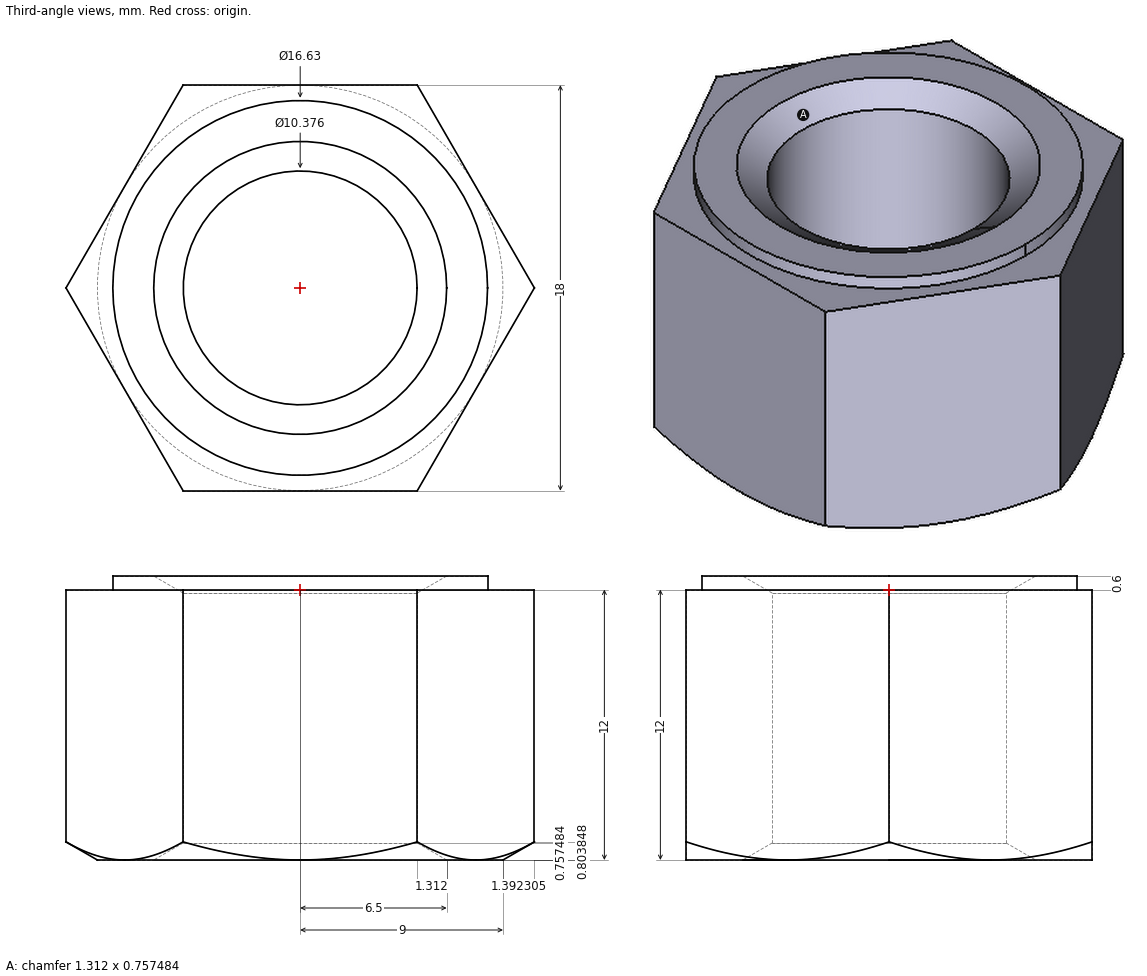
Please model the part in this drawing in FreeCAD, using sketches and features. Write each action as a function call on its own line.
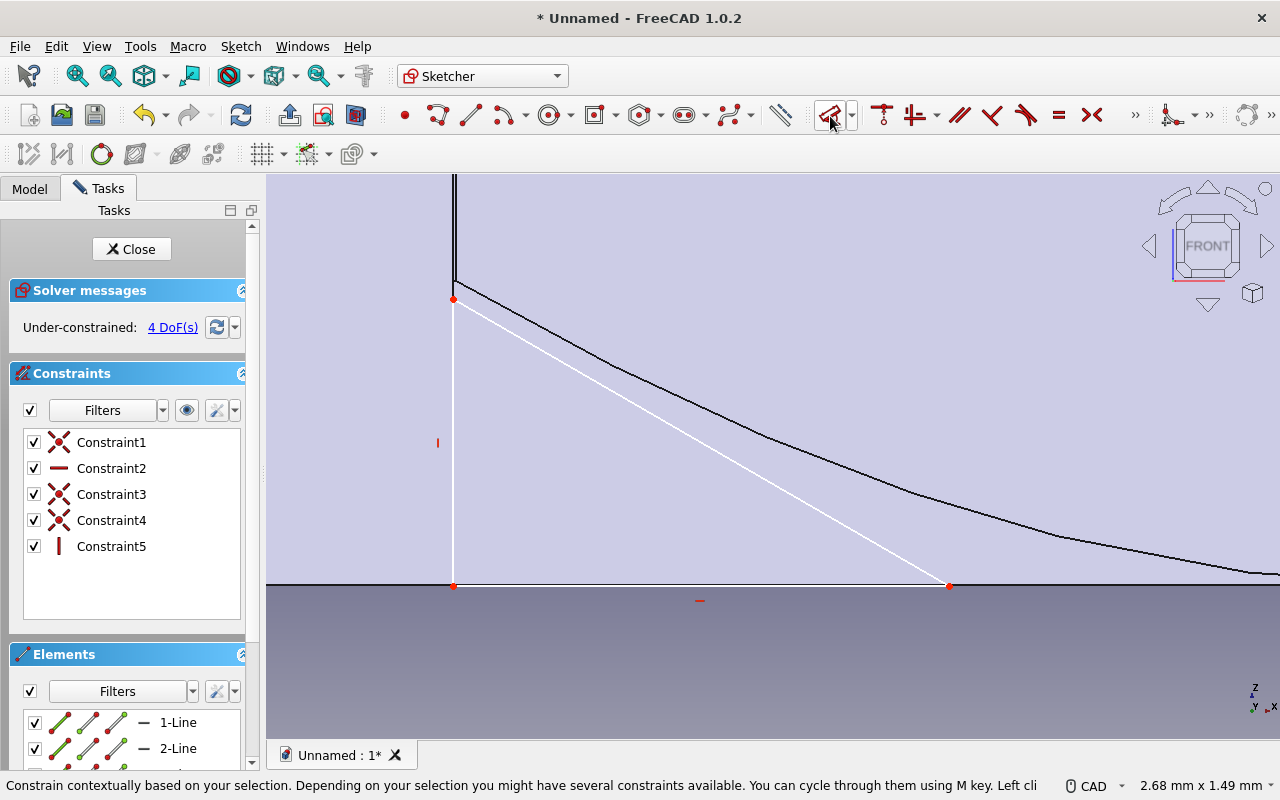
click(949, 586)
click(983, 394)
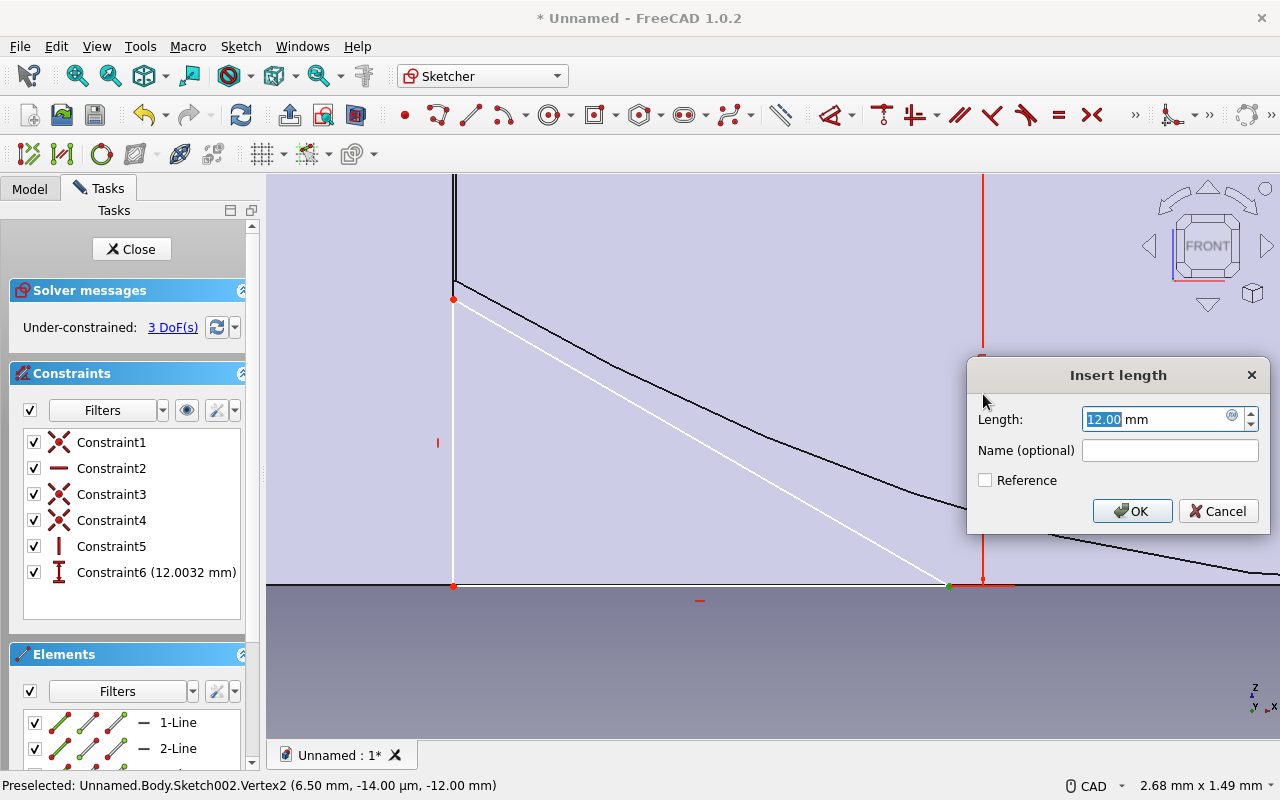
text(12)
key(Return)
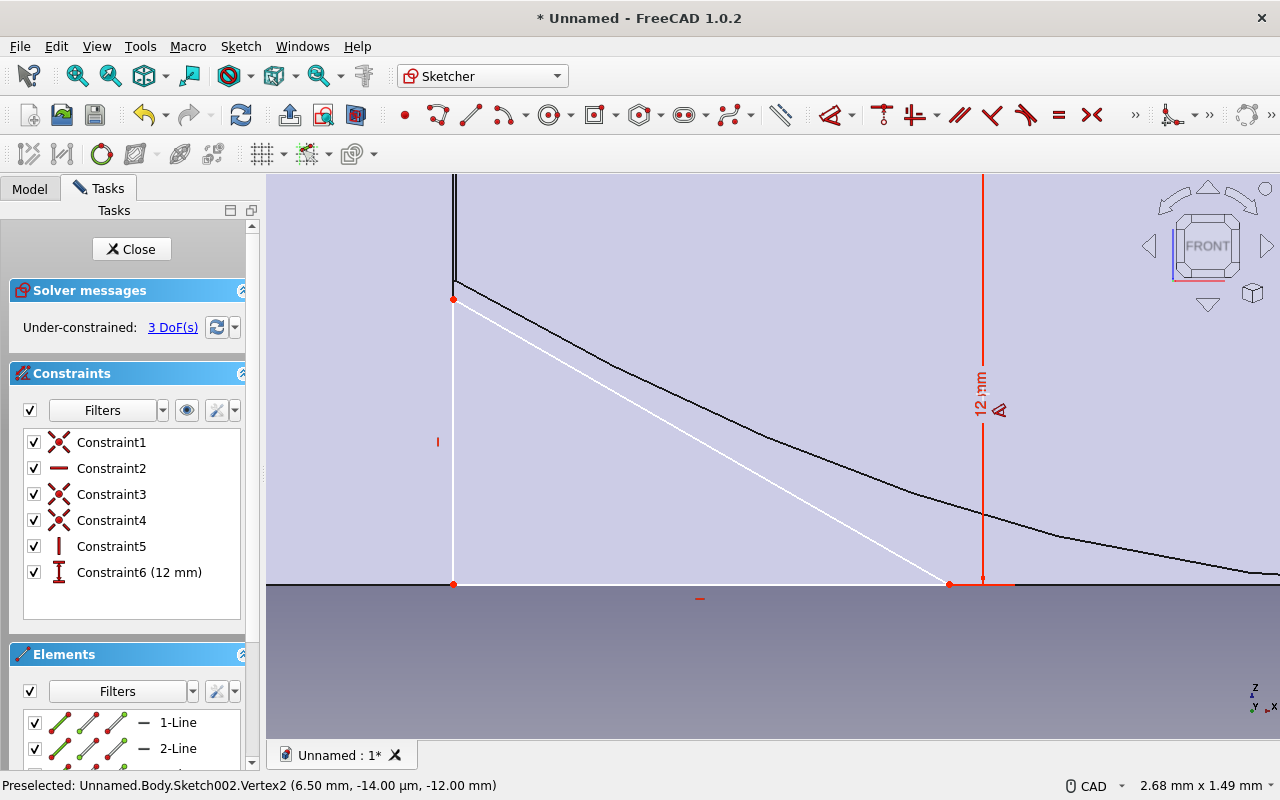
click(949, 585)
click(621, 619)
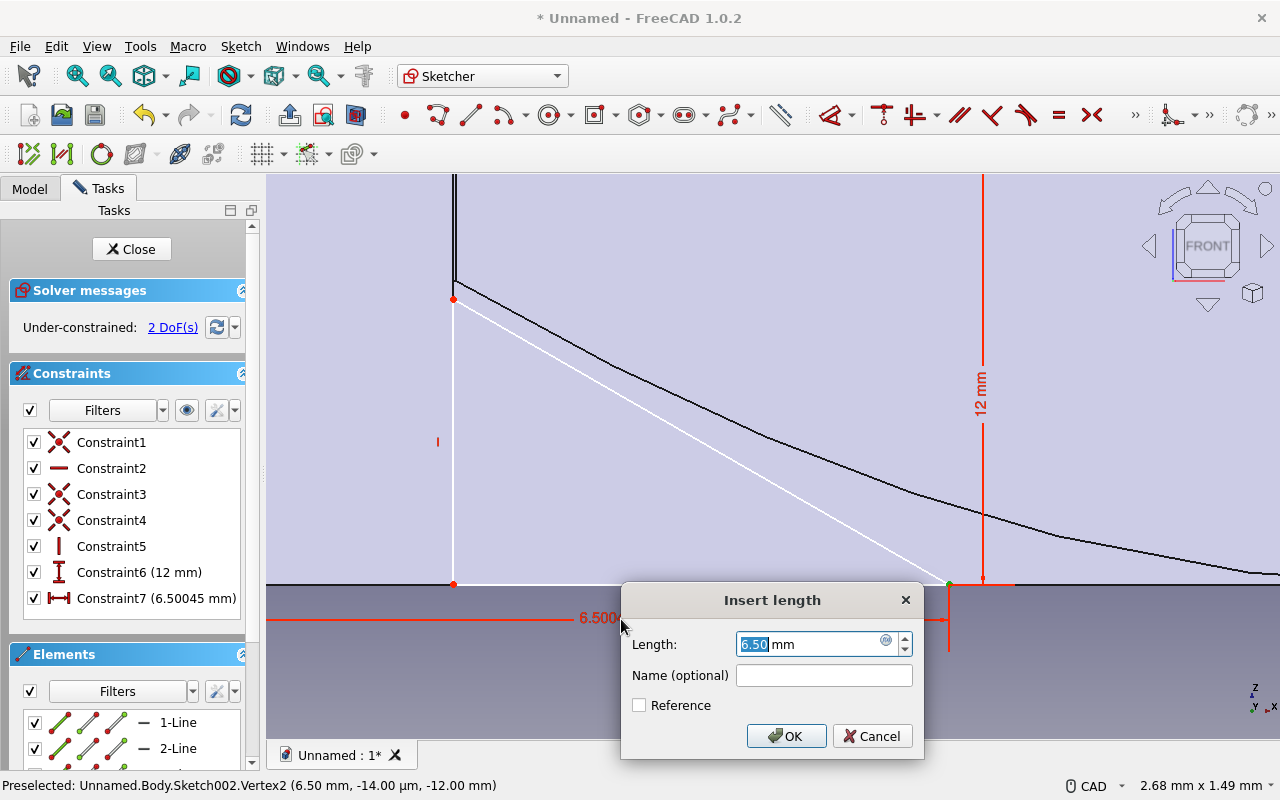
text(6.5)
key(Return)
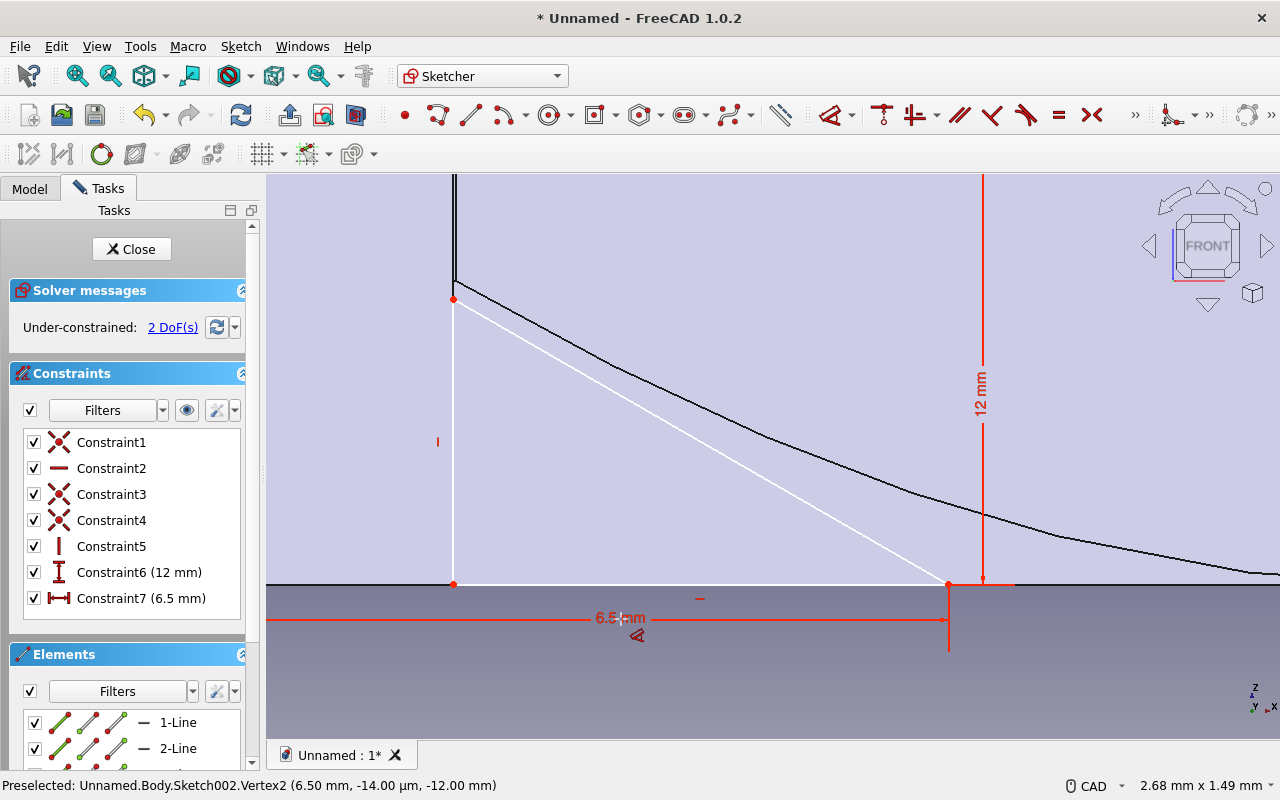
click(800, 585)
click(701, 619)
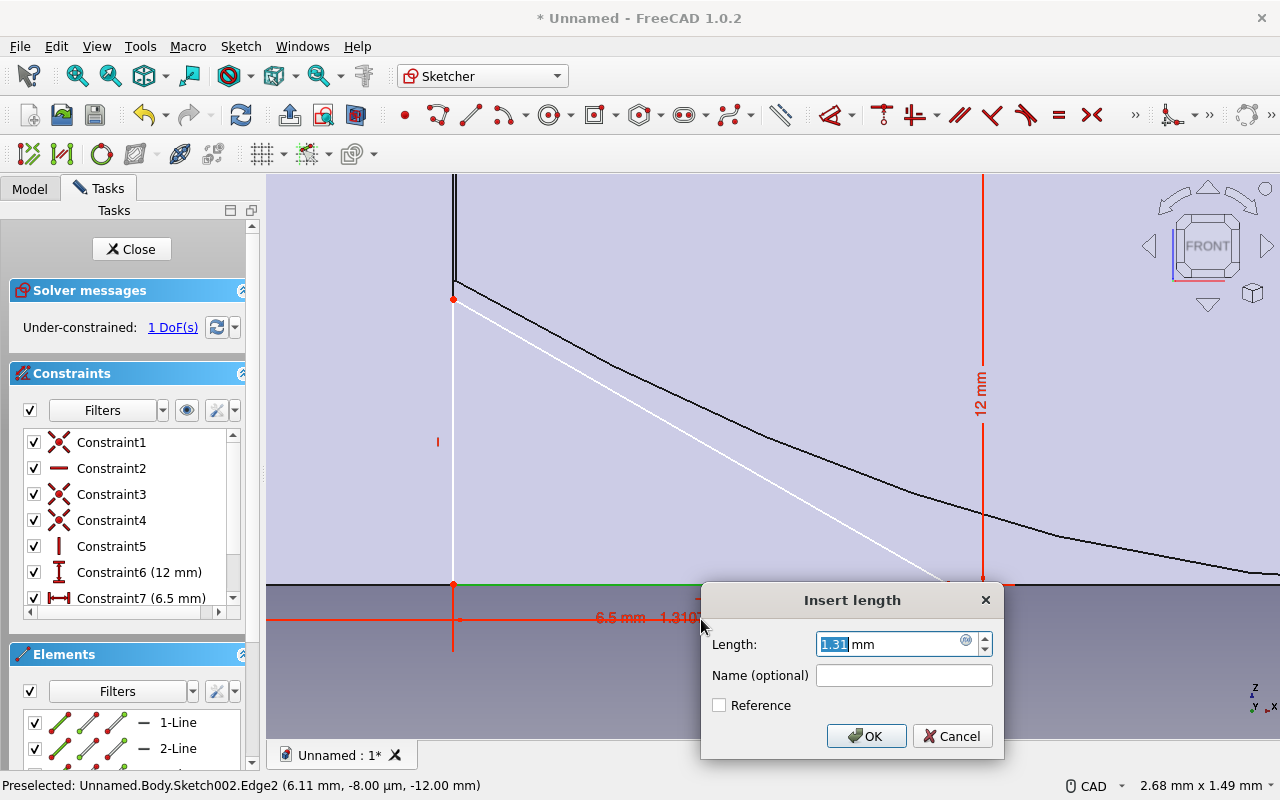
text(1.312)
key(Return)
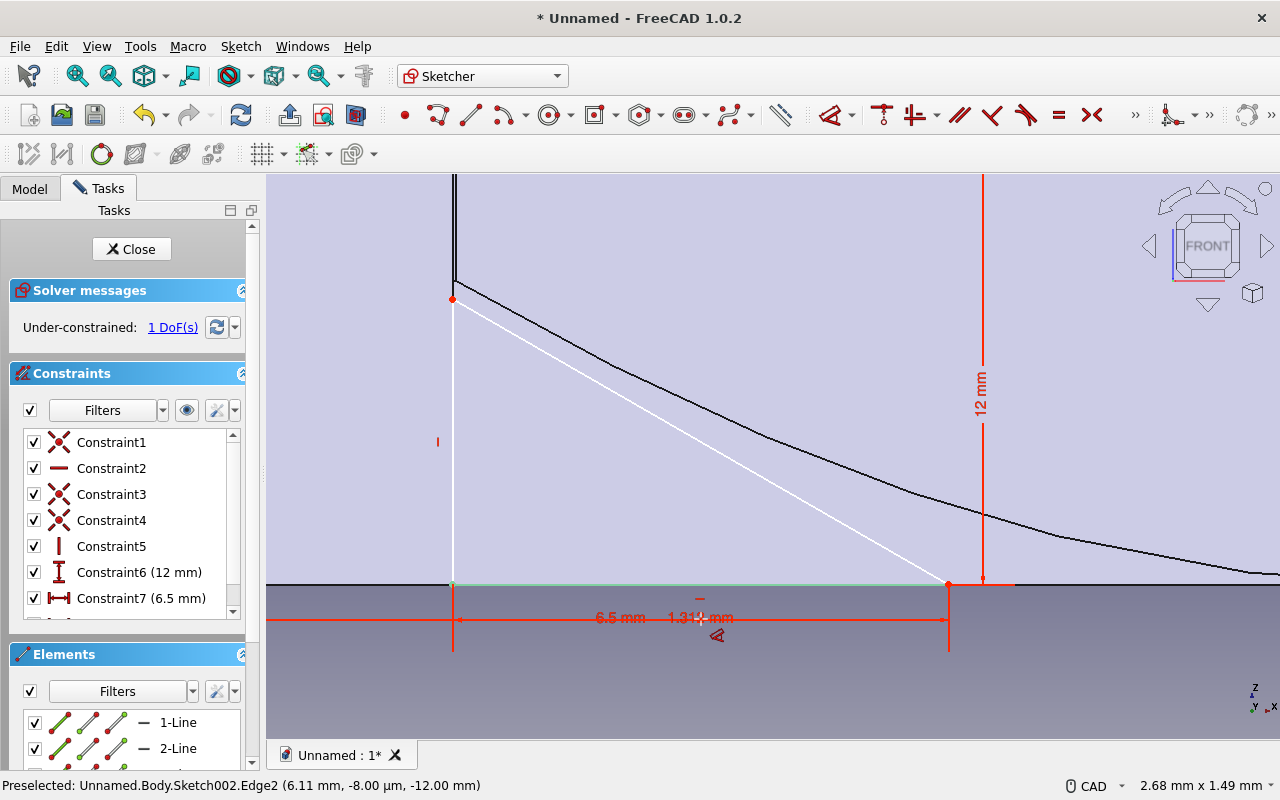
click(453, 499)
click(419, 442)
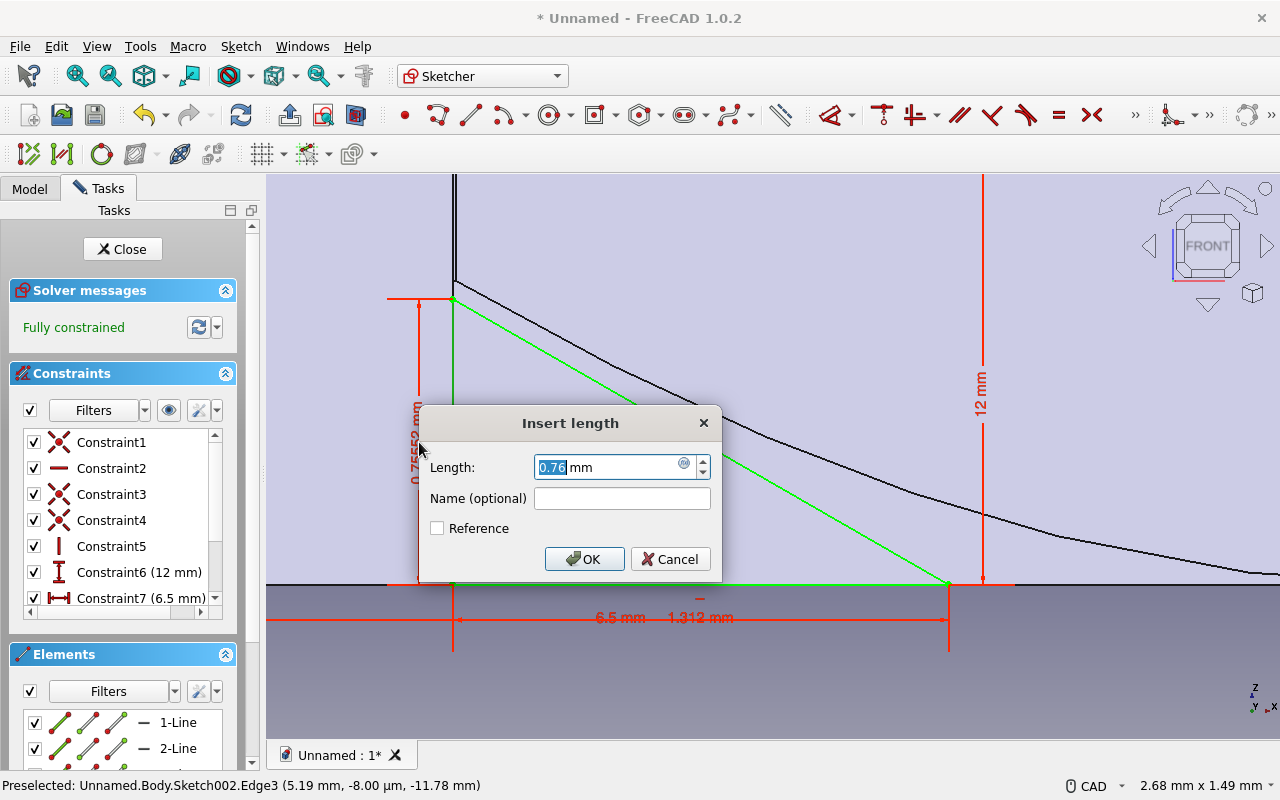
text(0.757484)
key(Return)
key(Escape)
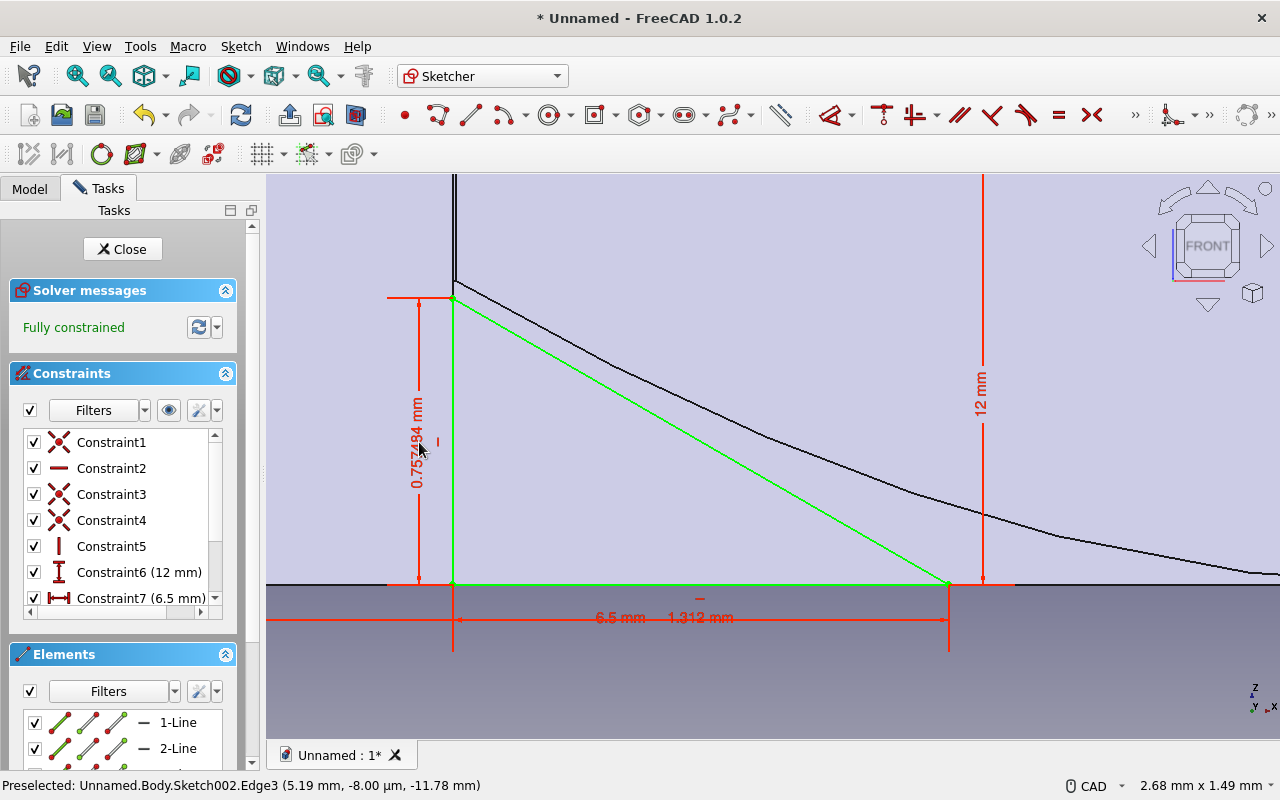
click(123, 249)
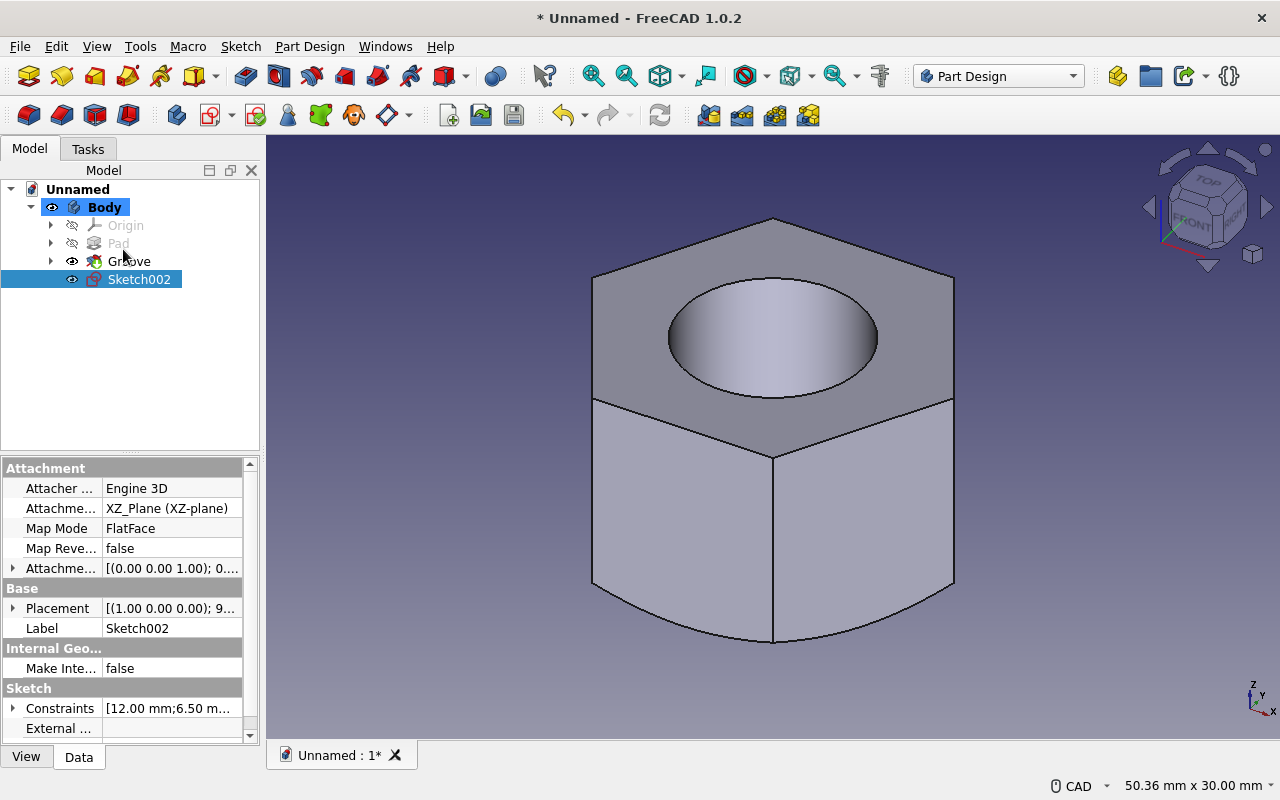
click(312, 76)